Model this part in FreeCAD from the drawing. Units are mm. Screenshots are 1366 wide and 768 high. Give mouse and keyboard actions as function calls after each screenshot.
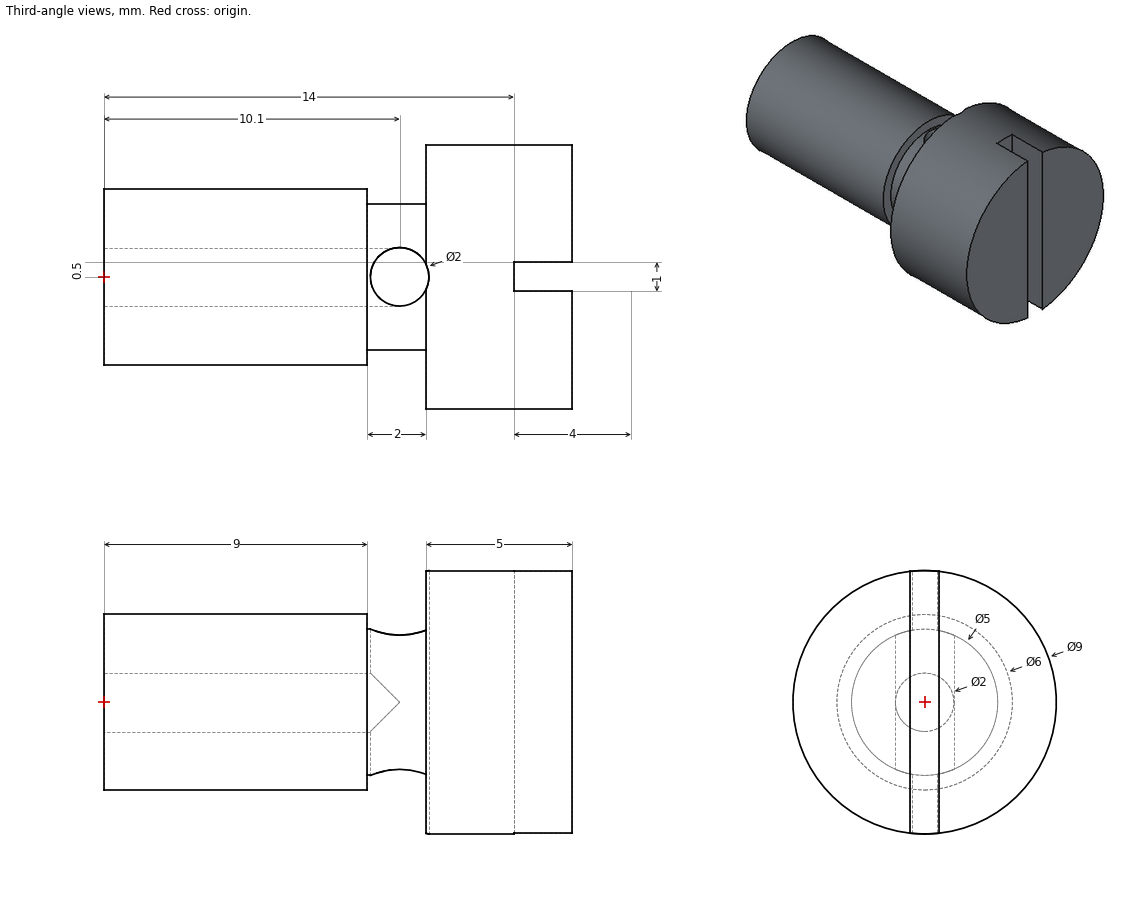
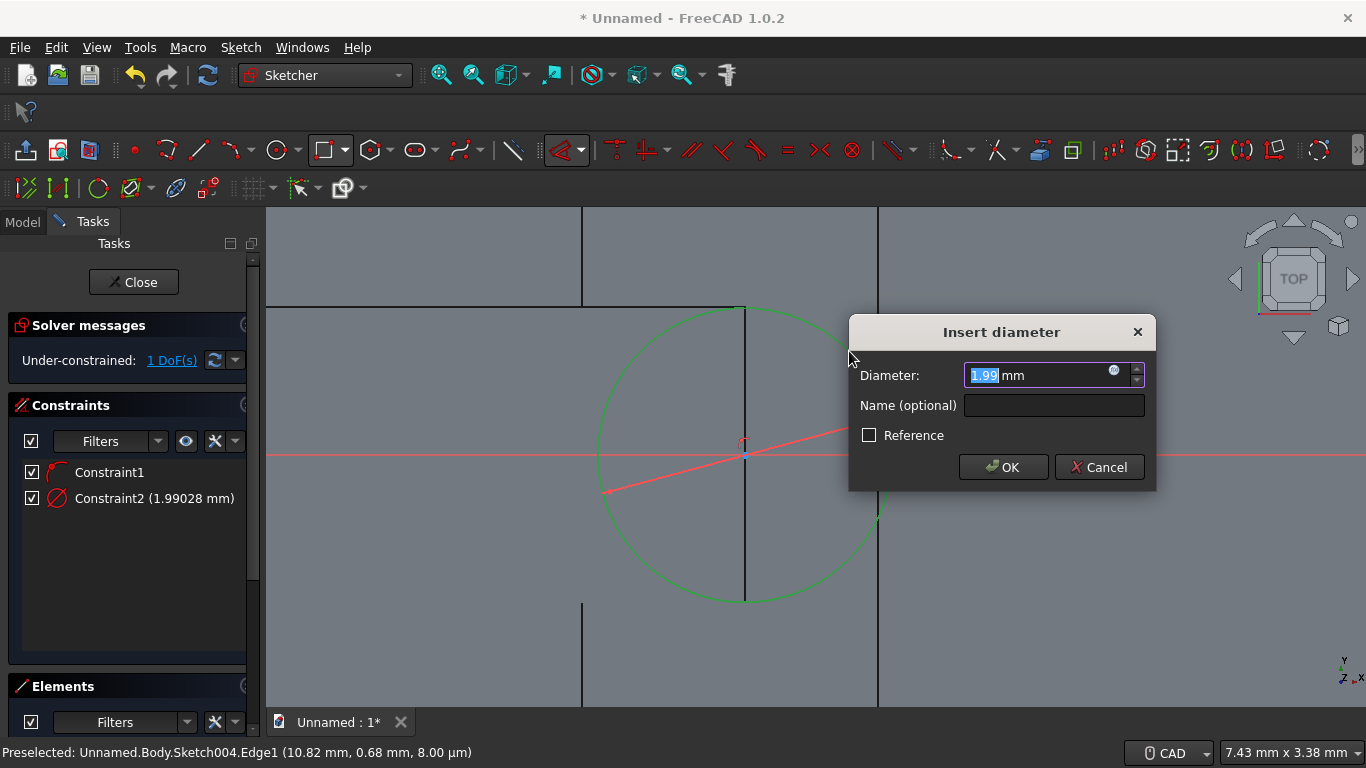
text(2)
key(Return)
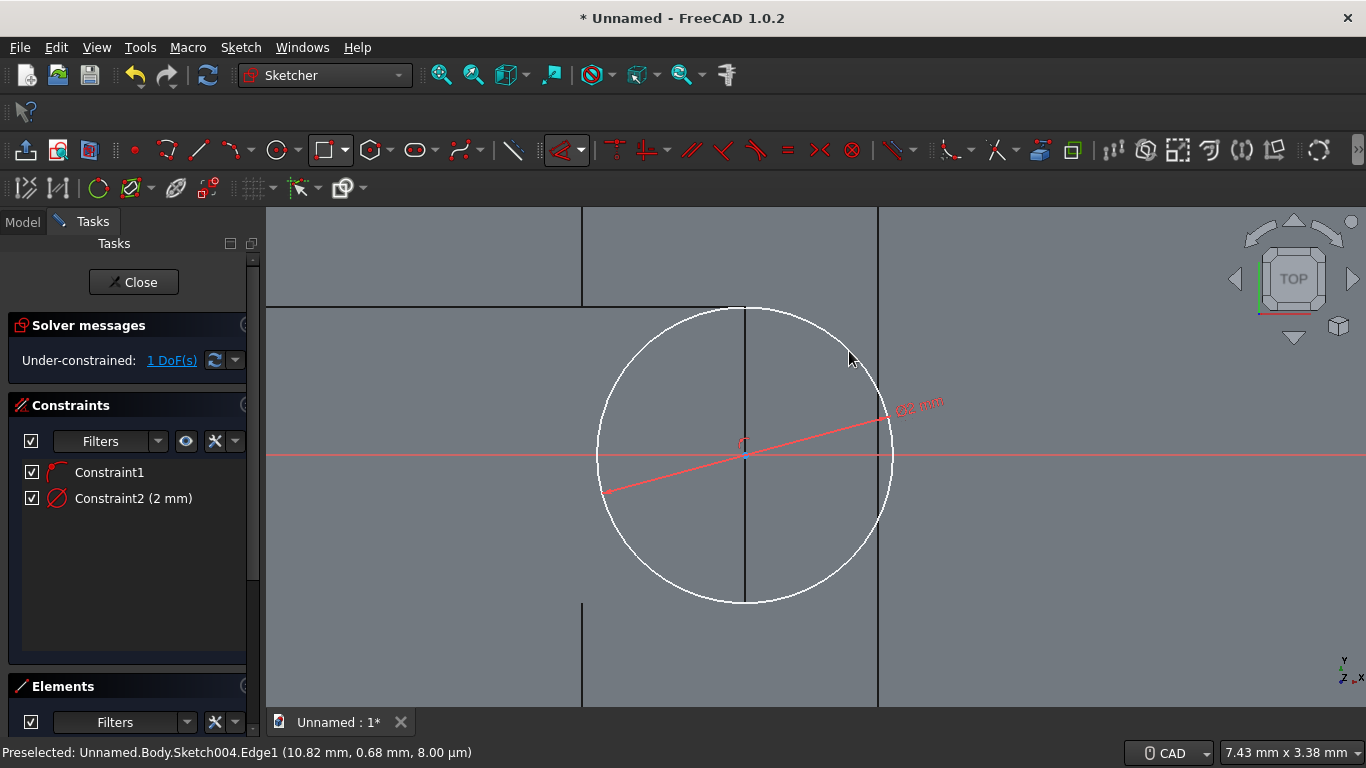
click(745, 455)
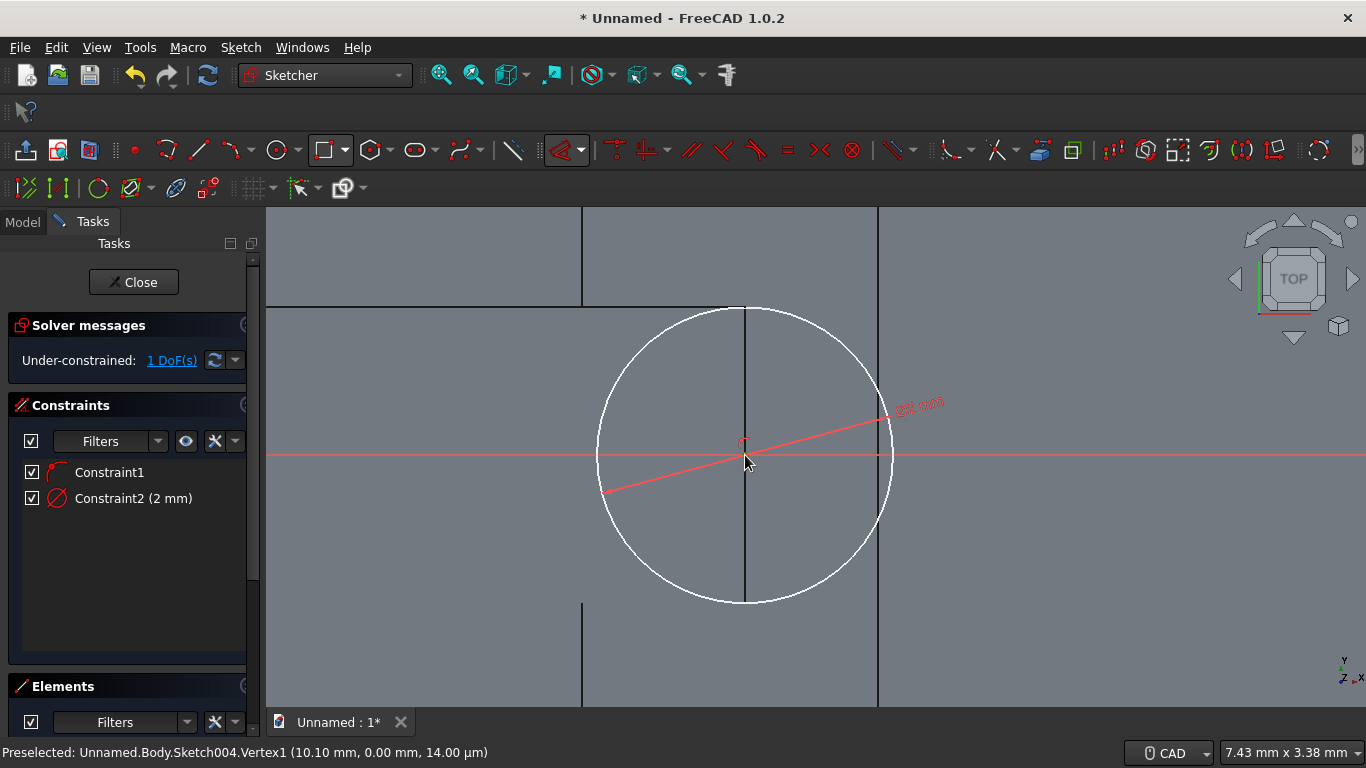
click(584, 150)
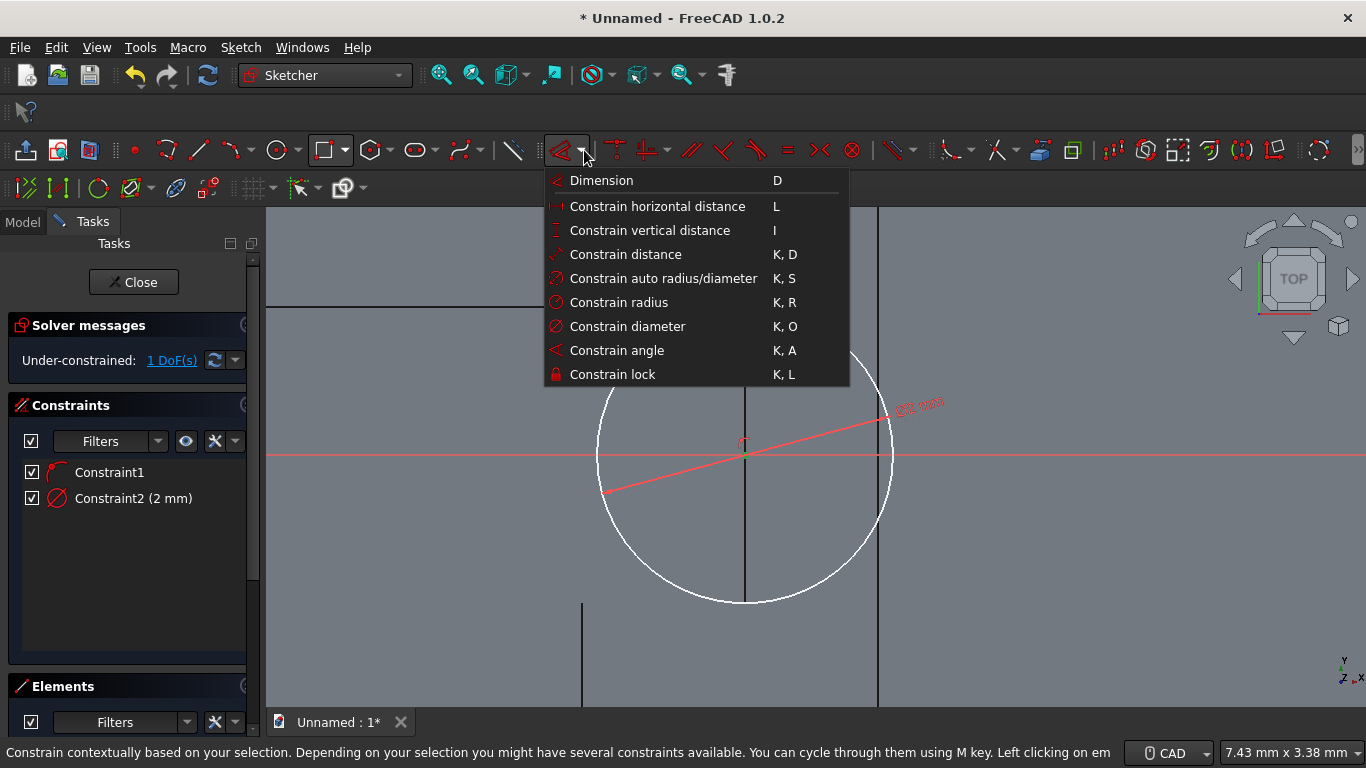
click(697, 206)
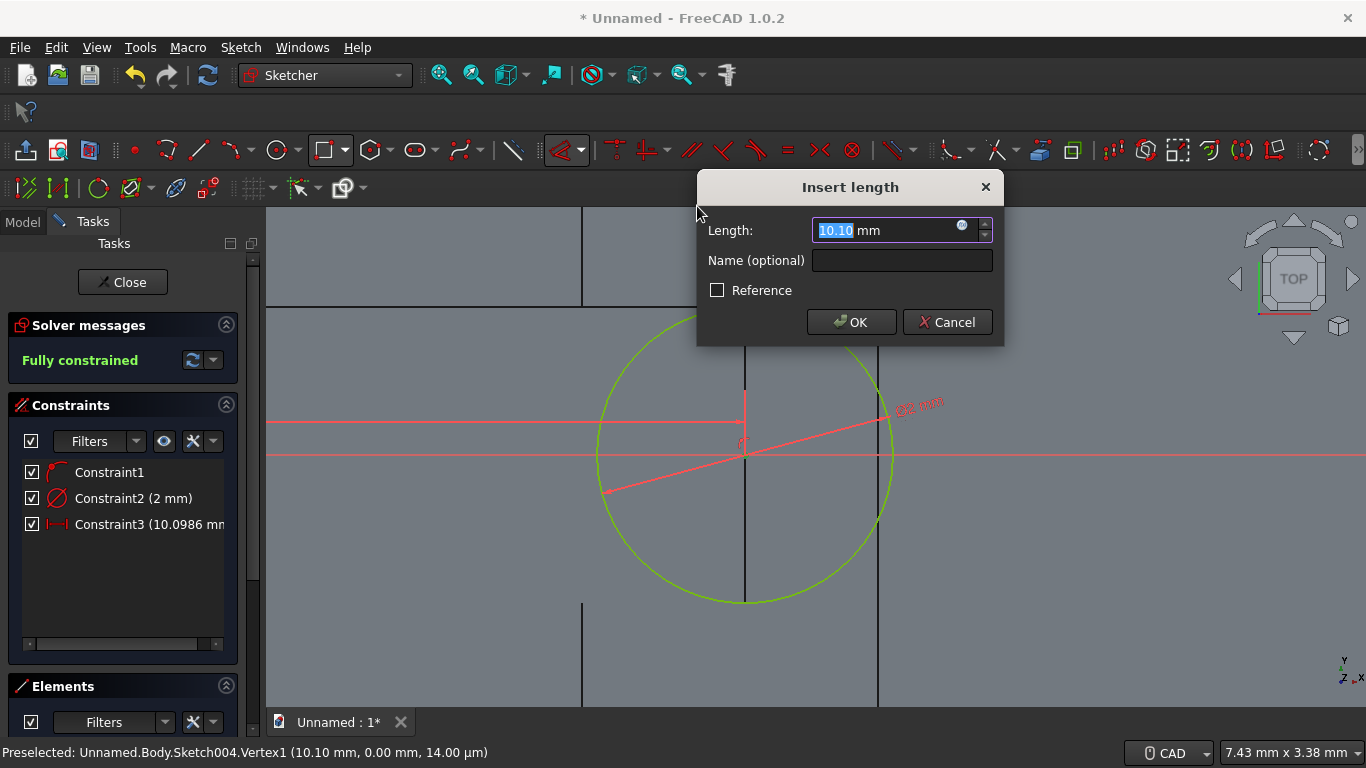
text(10.1)
key(Return)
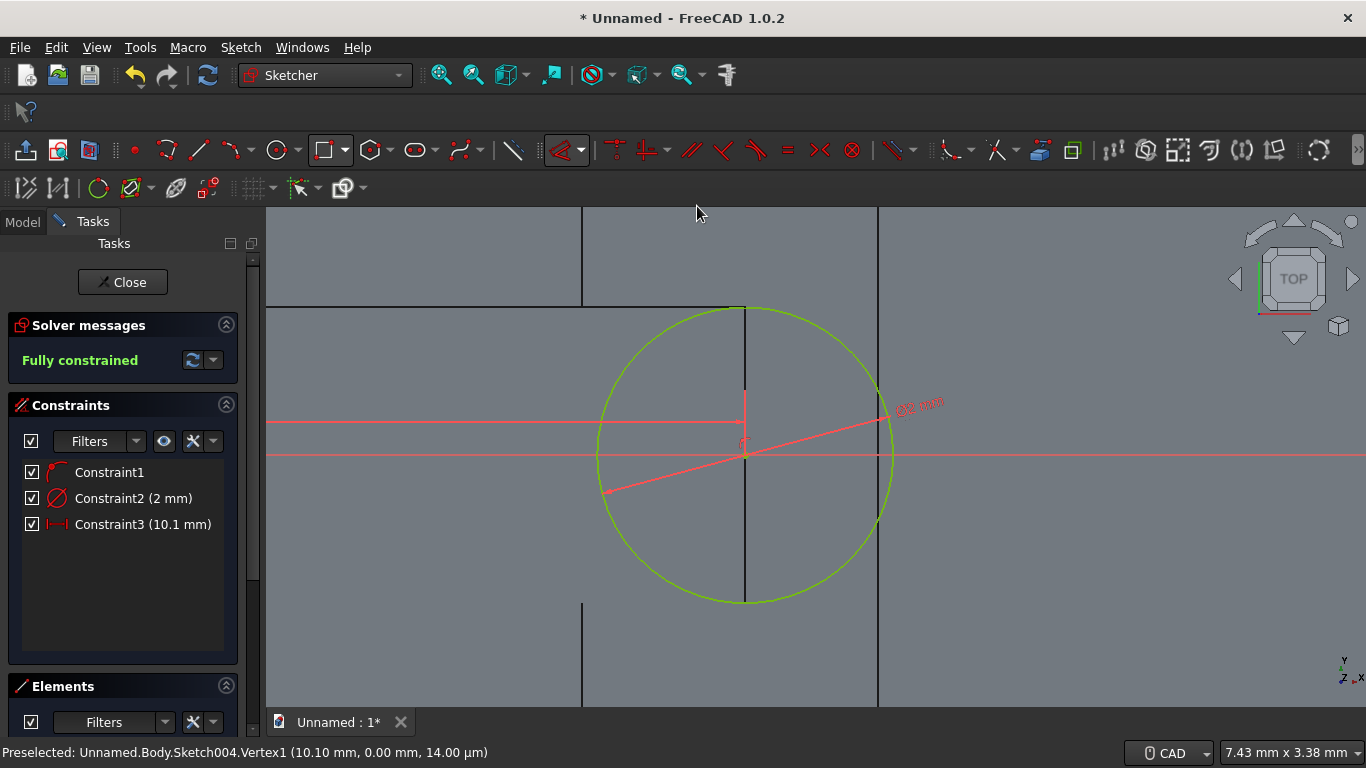
click(123, 282)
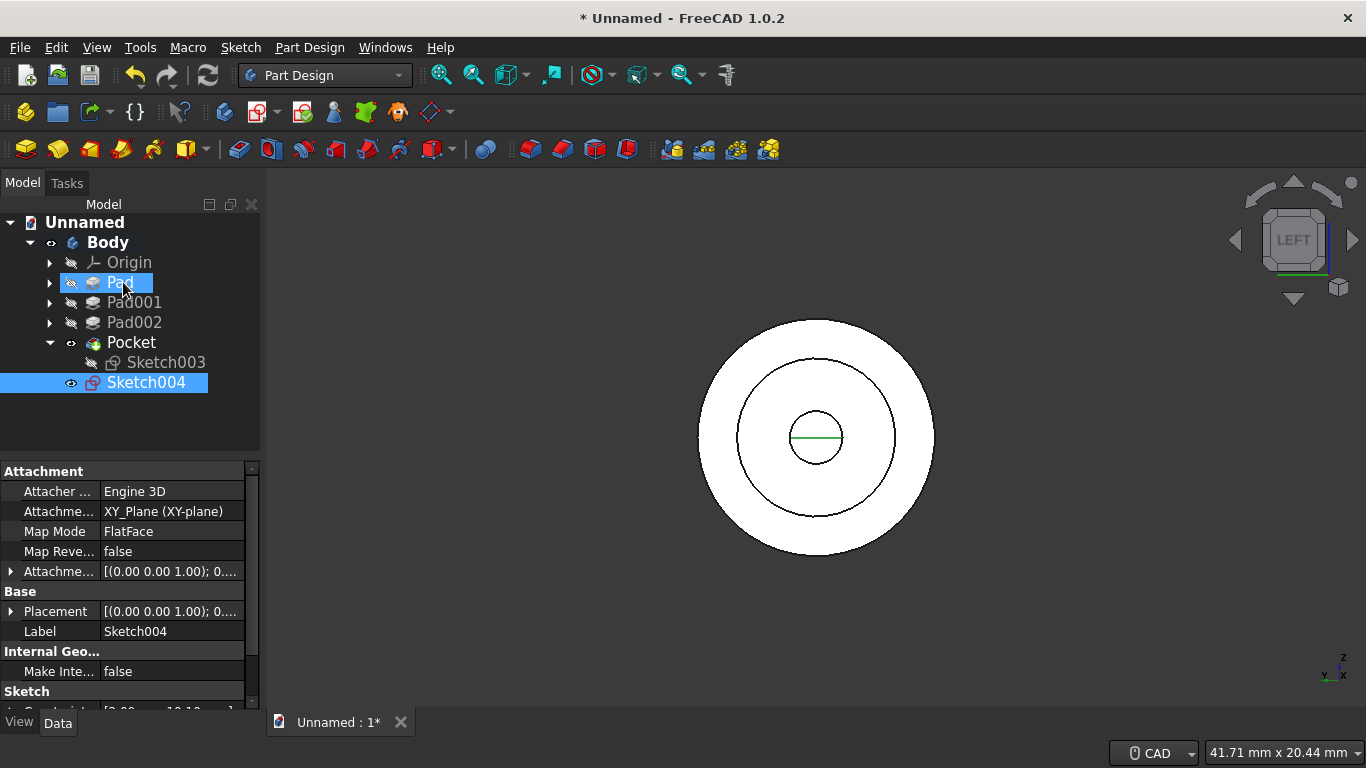
click(240, 150)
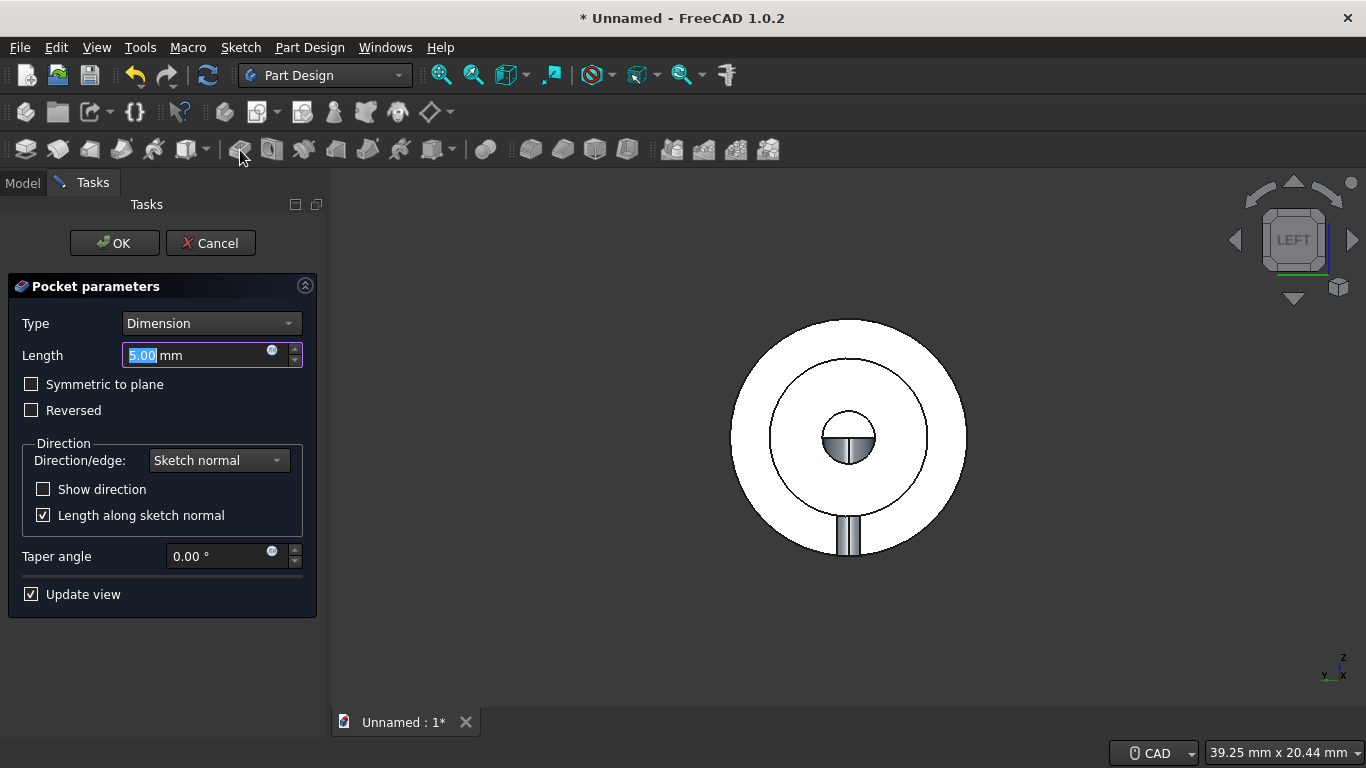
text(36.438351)
key(Tab)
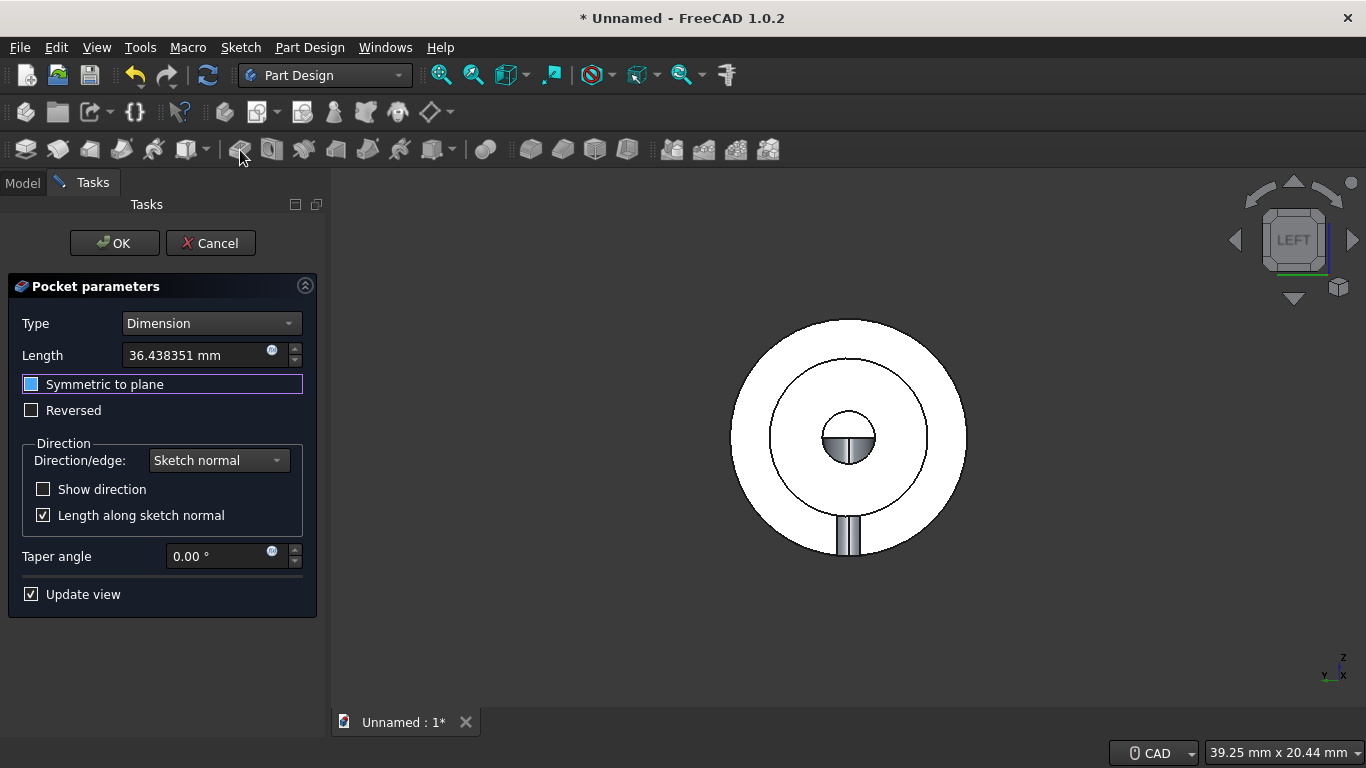
click(30, 384)